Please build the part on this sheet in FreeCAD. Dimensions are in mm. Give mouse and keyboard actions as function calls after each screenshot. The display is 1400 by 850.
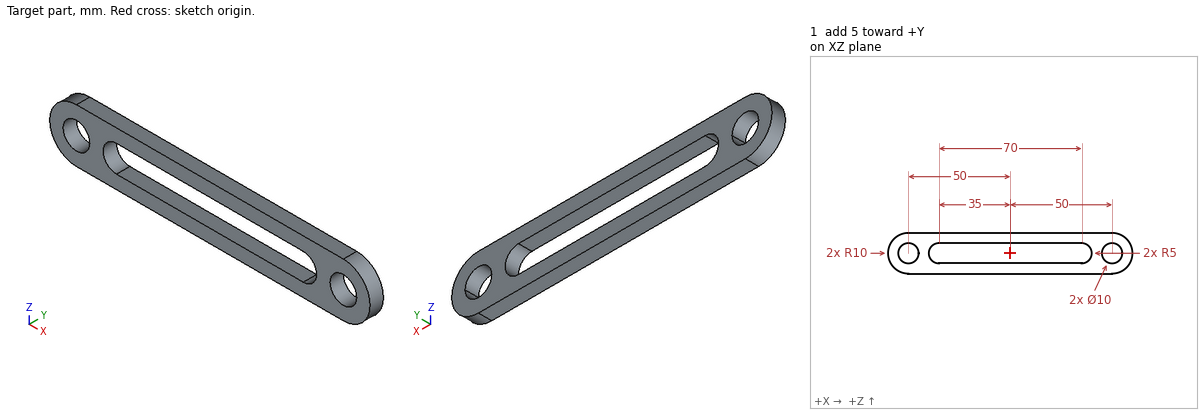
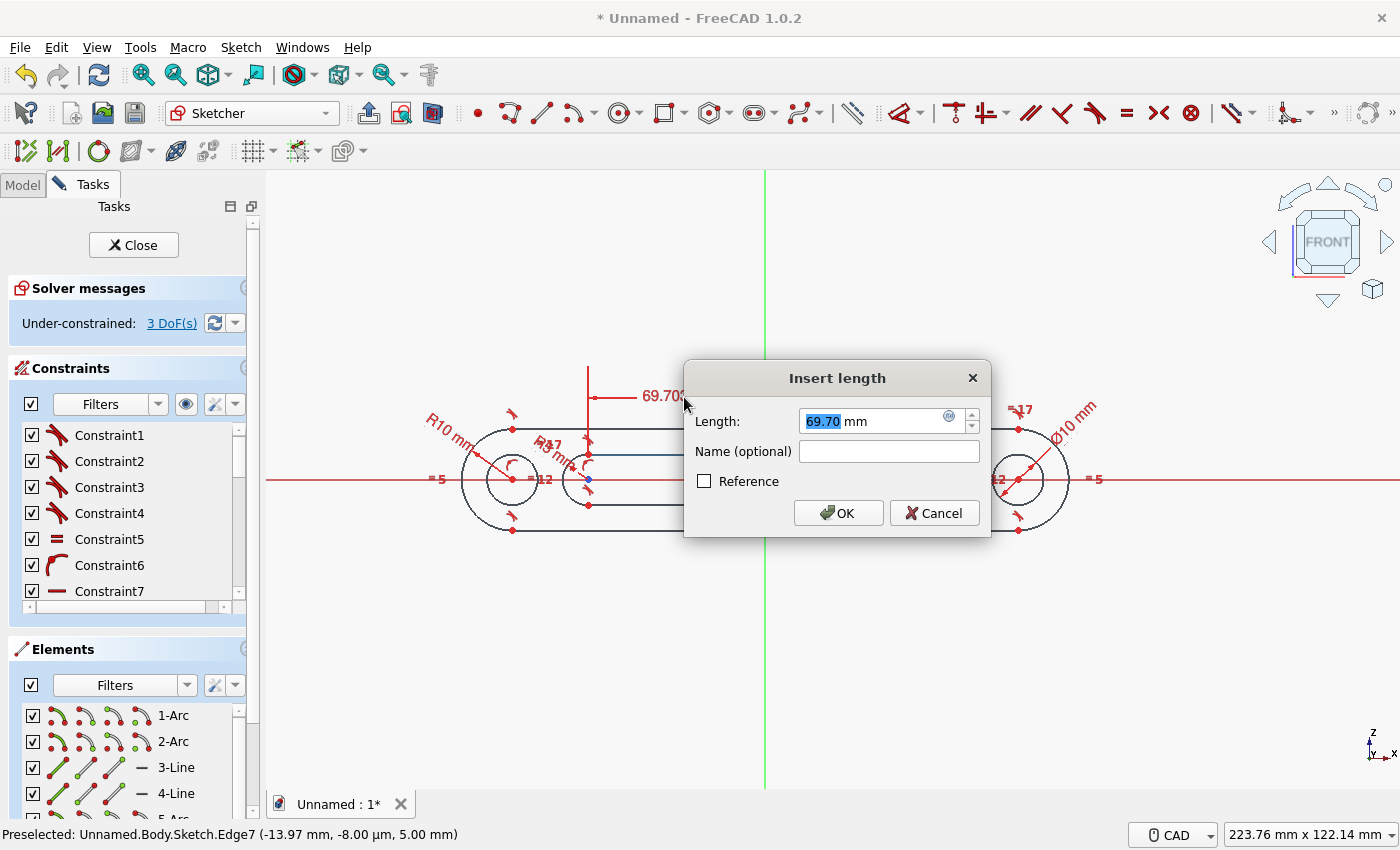
text(70)
key(Return)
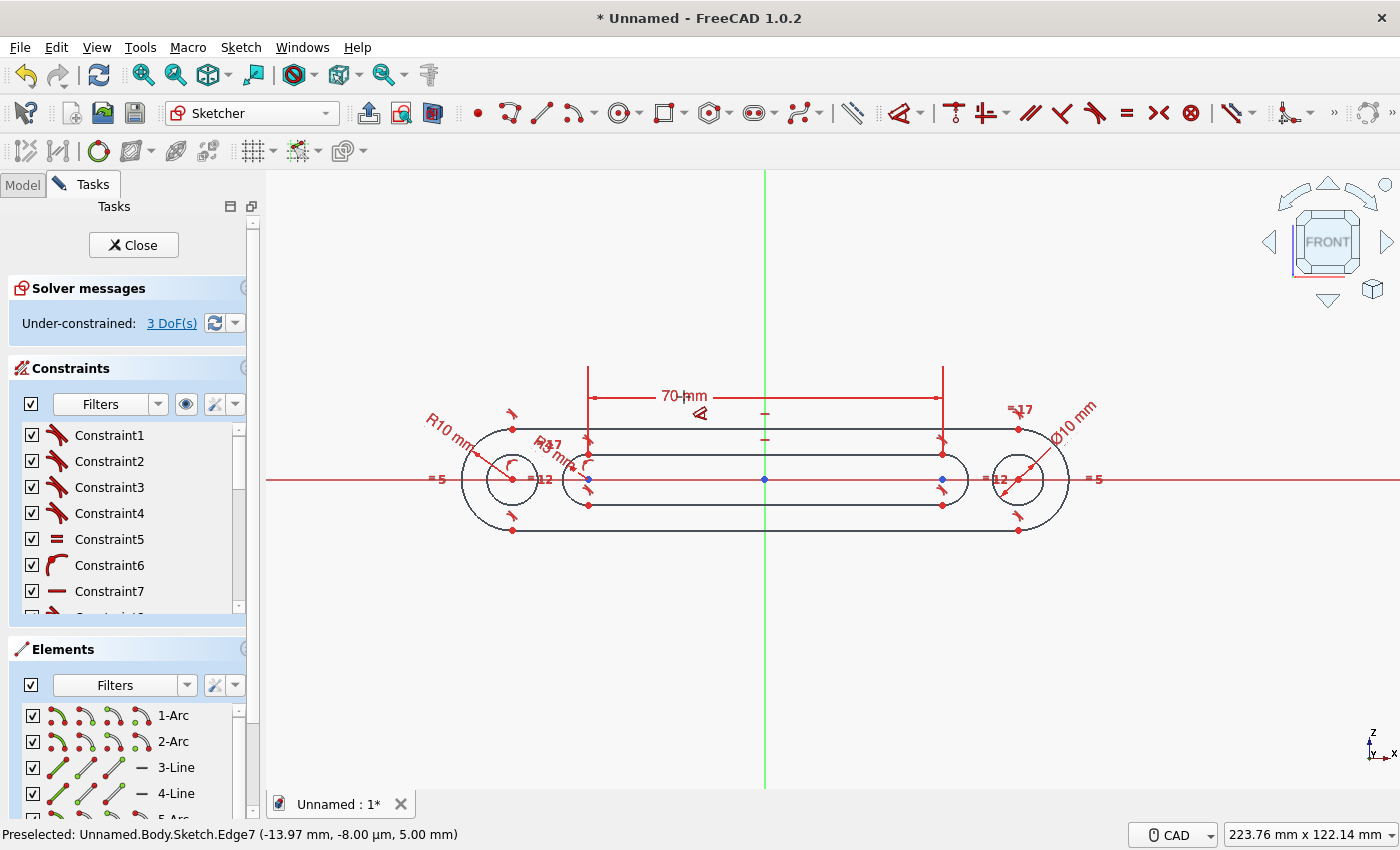
click(1018, 480)
click(980, 514)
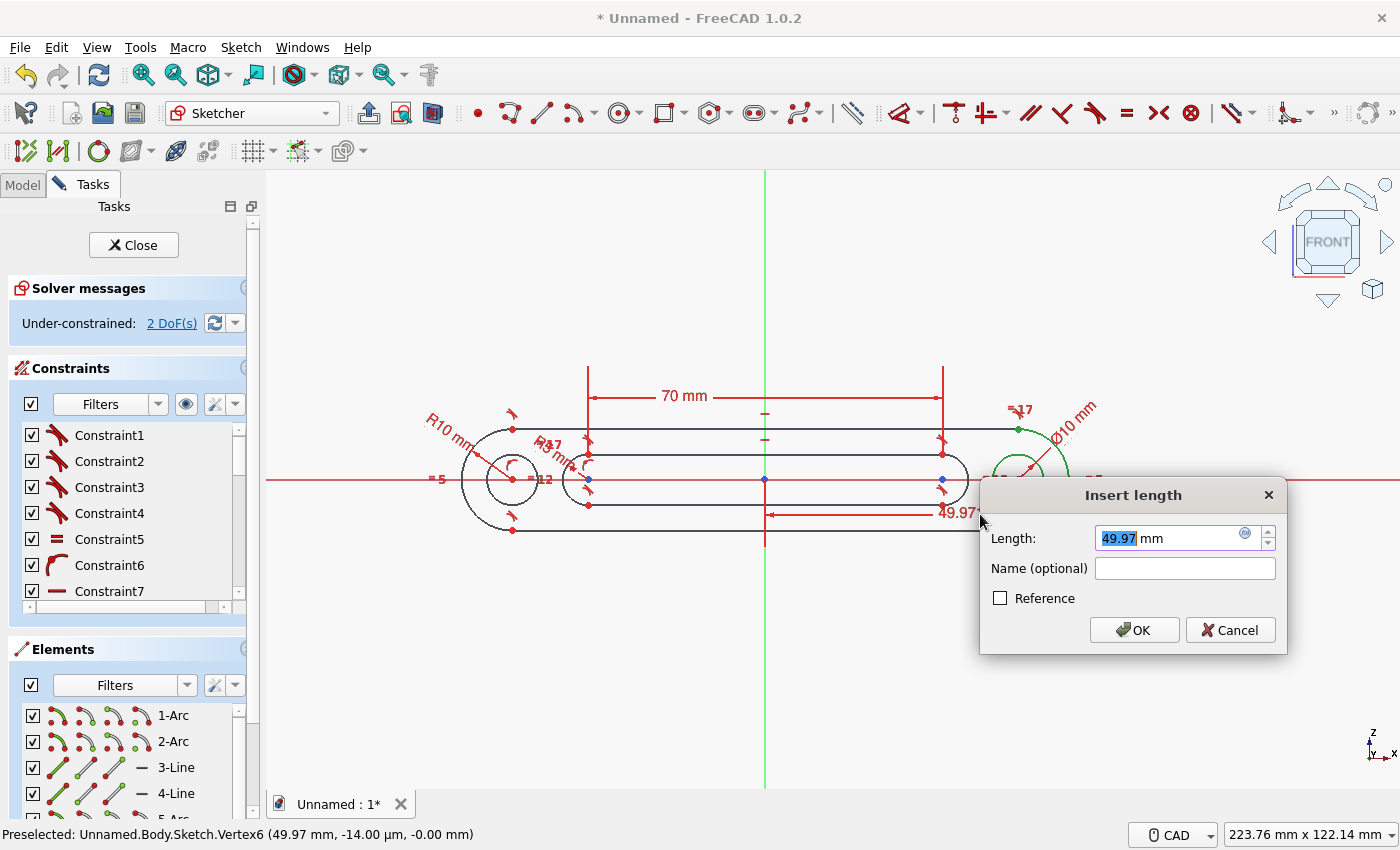
text(50)
key(Return)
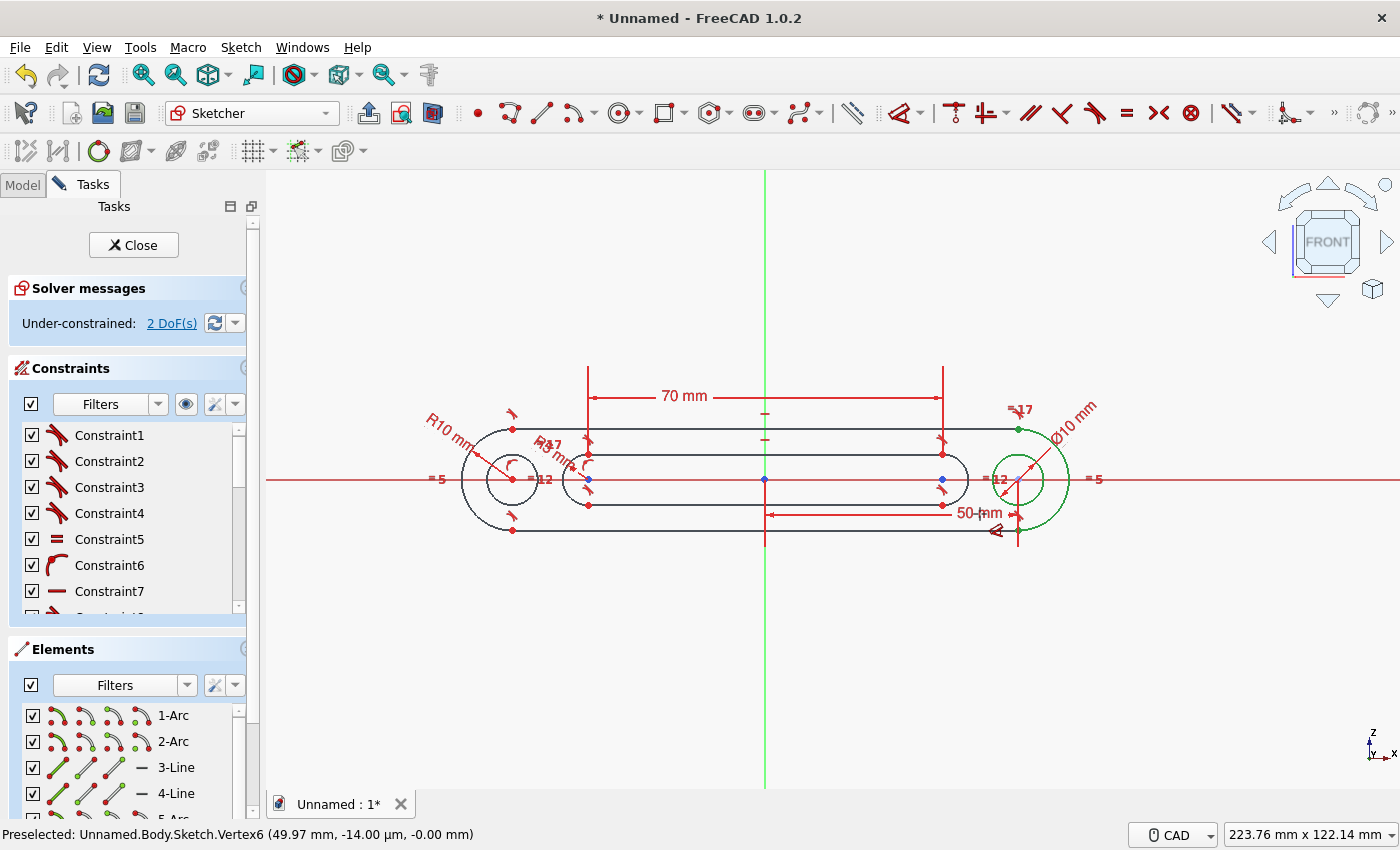
click(512, 480)
click(550, 514)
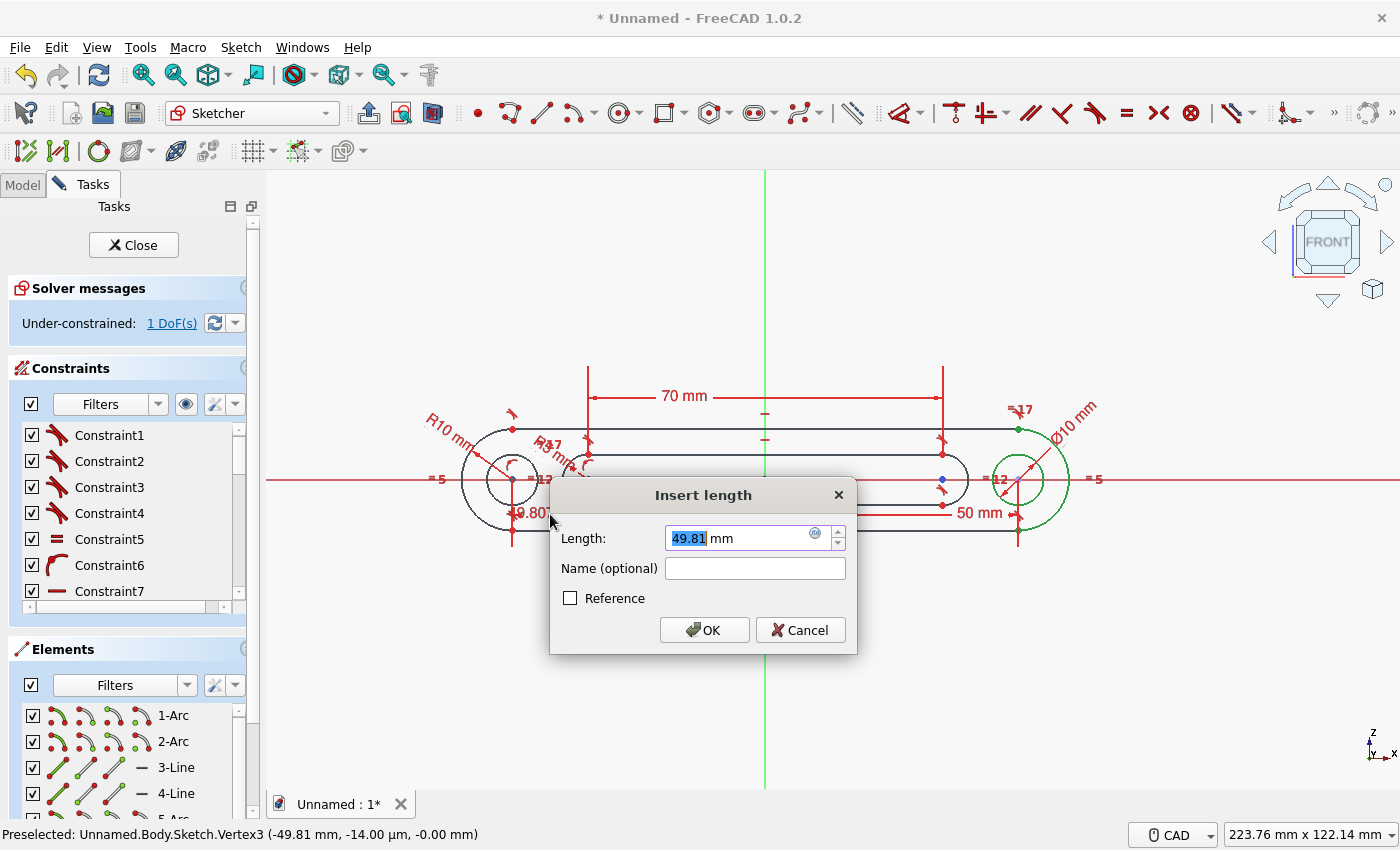
text(50)
key(Return)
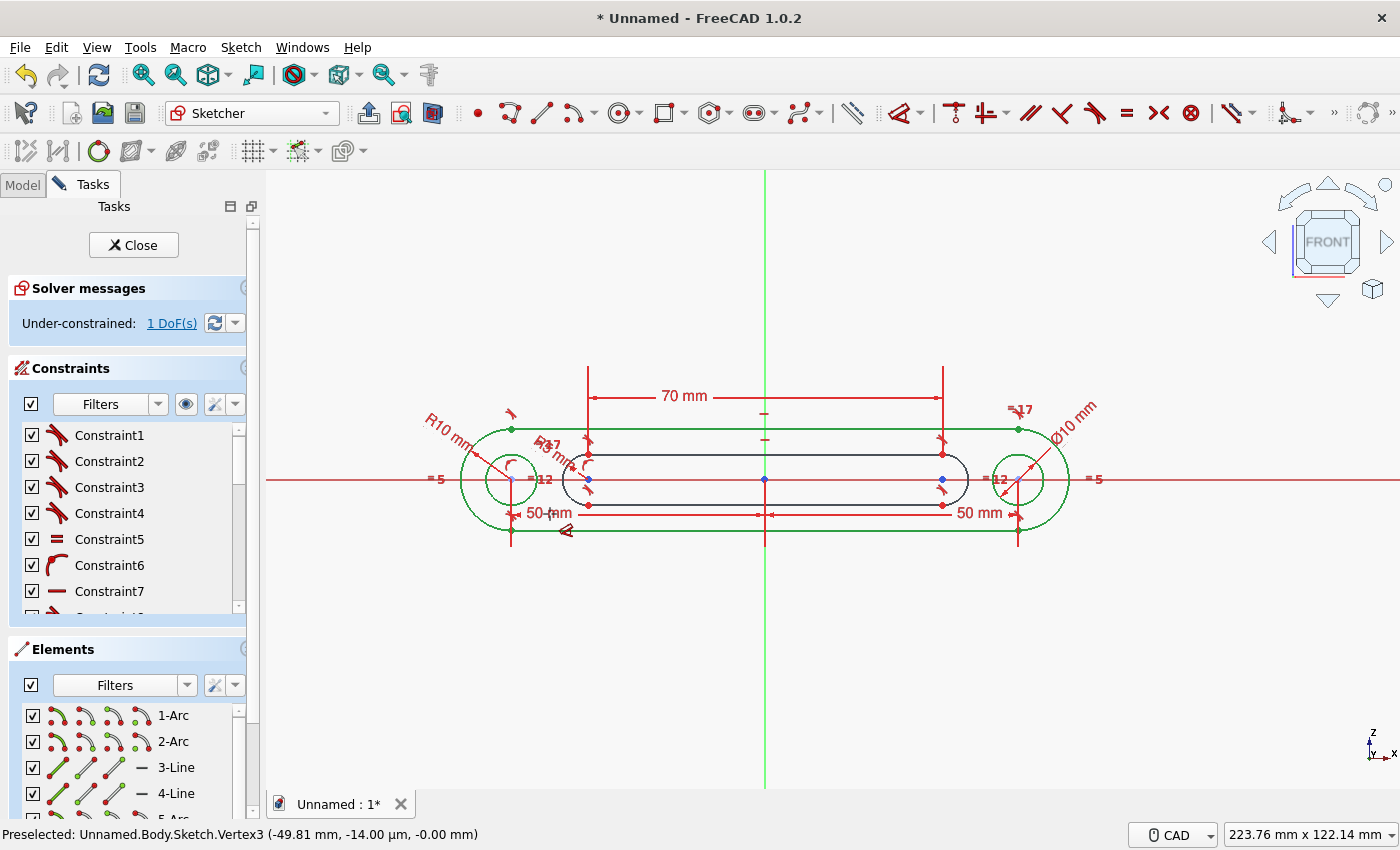
click(588, 455)
click(676, 373)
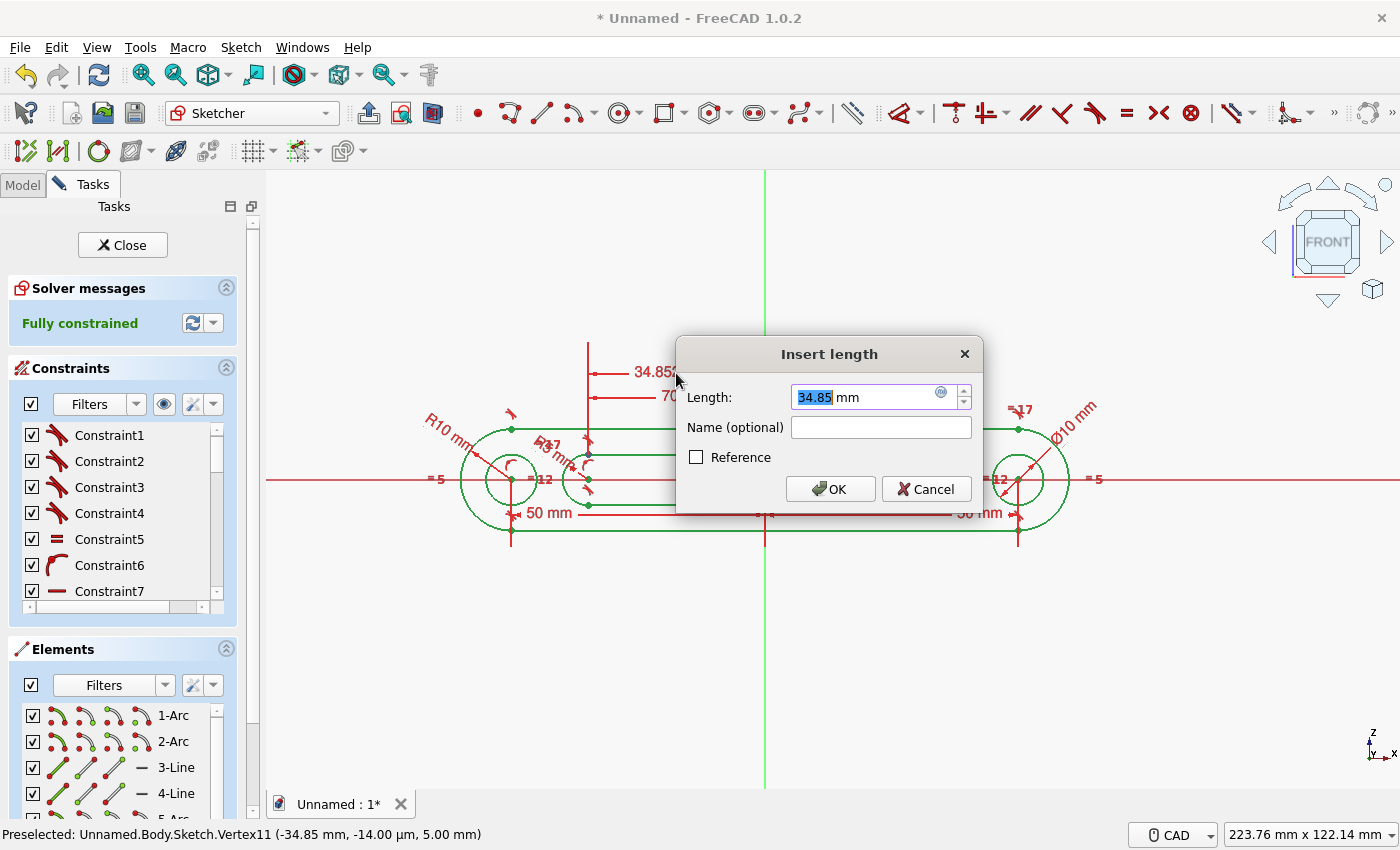
text(35)
key(Return)
key(Escape)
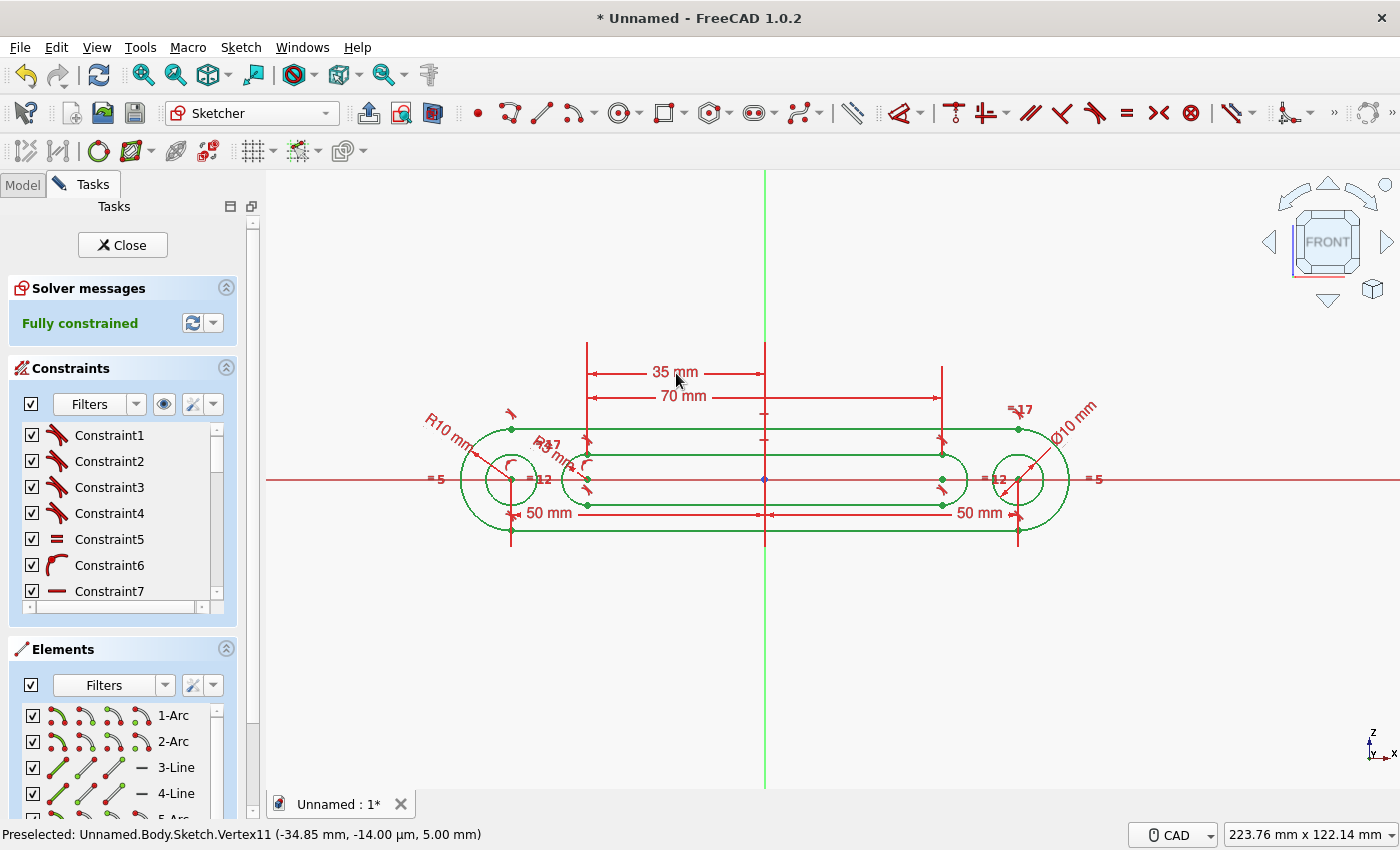
click(123, 245)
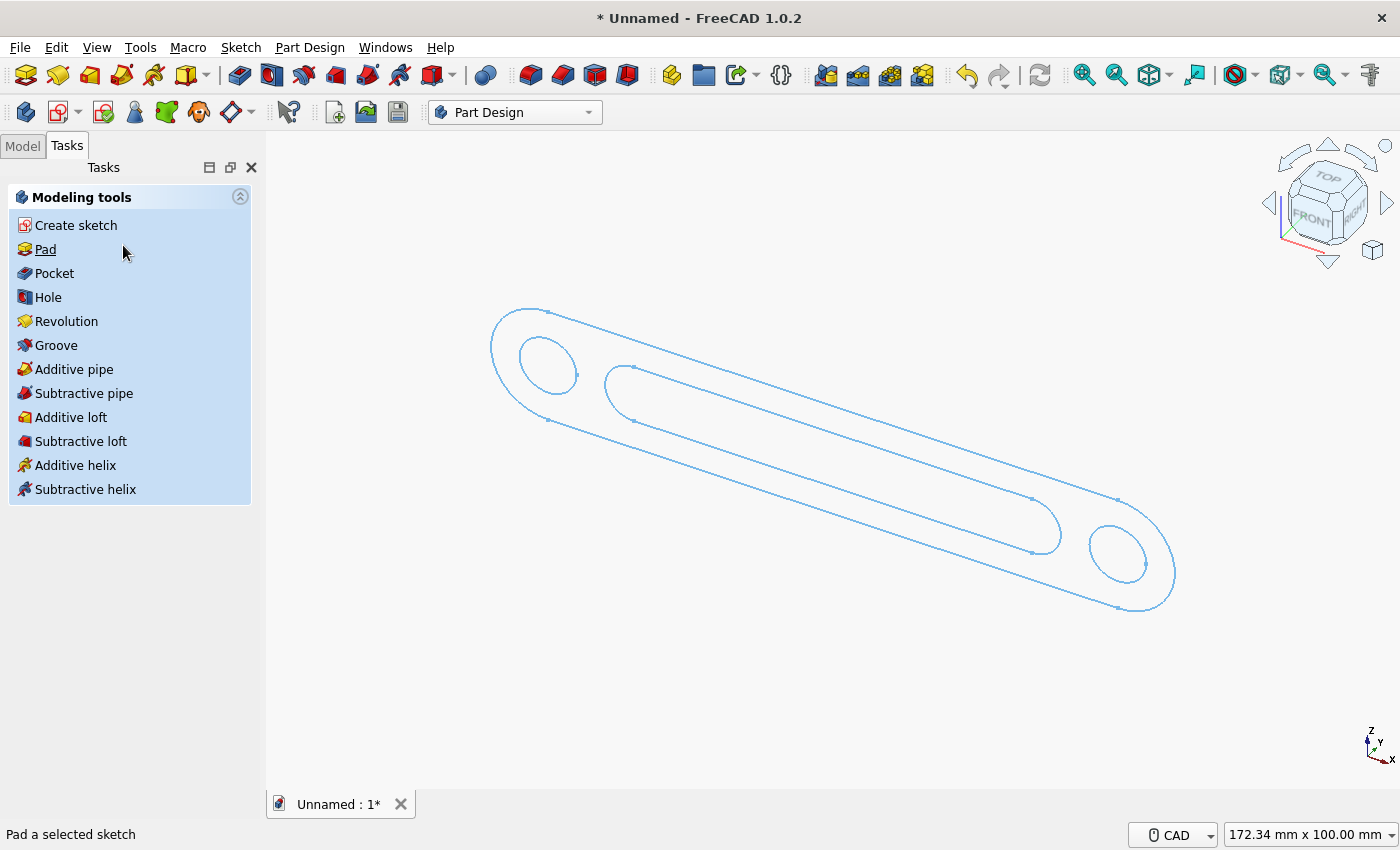
click(26, 76)